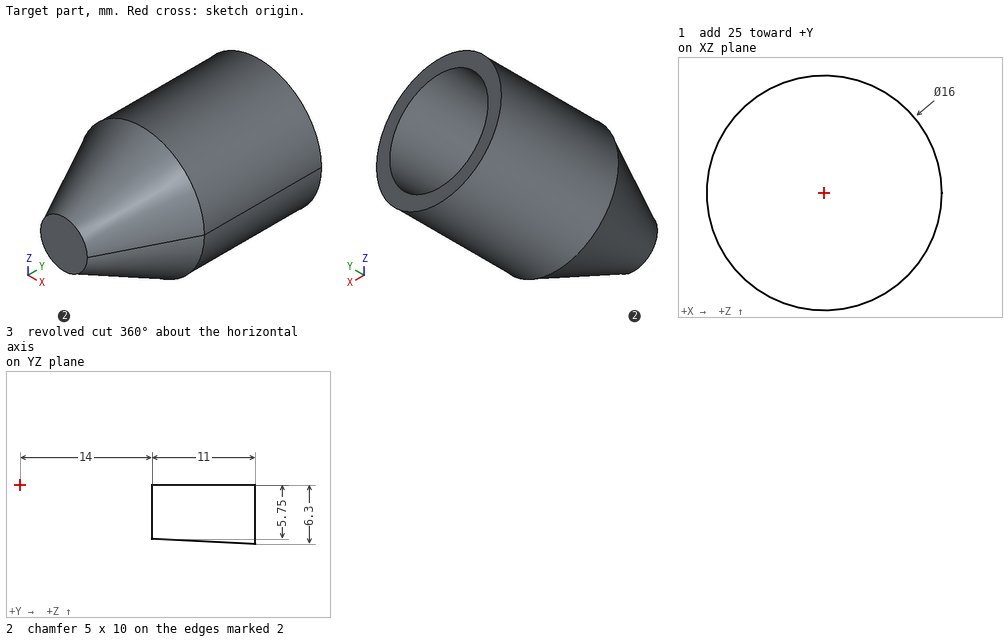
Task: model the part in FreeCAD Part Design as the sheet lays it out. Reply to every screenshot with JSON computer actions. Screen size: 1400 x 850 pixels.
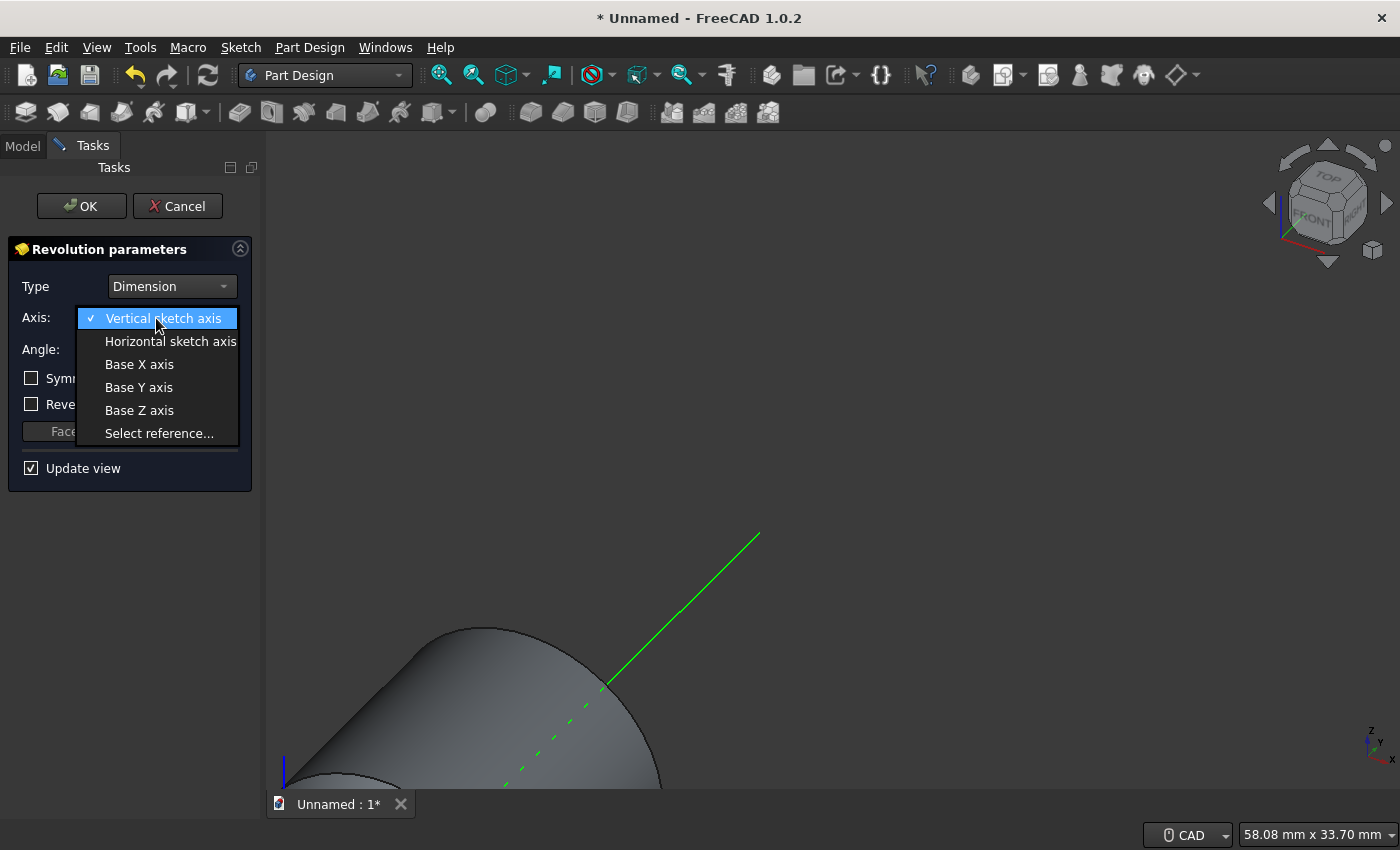
{"action": "left_click", "coordinate": [156, 342]}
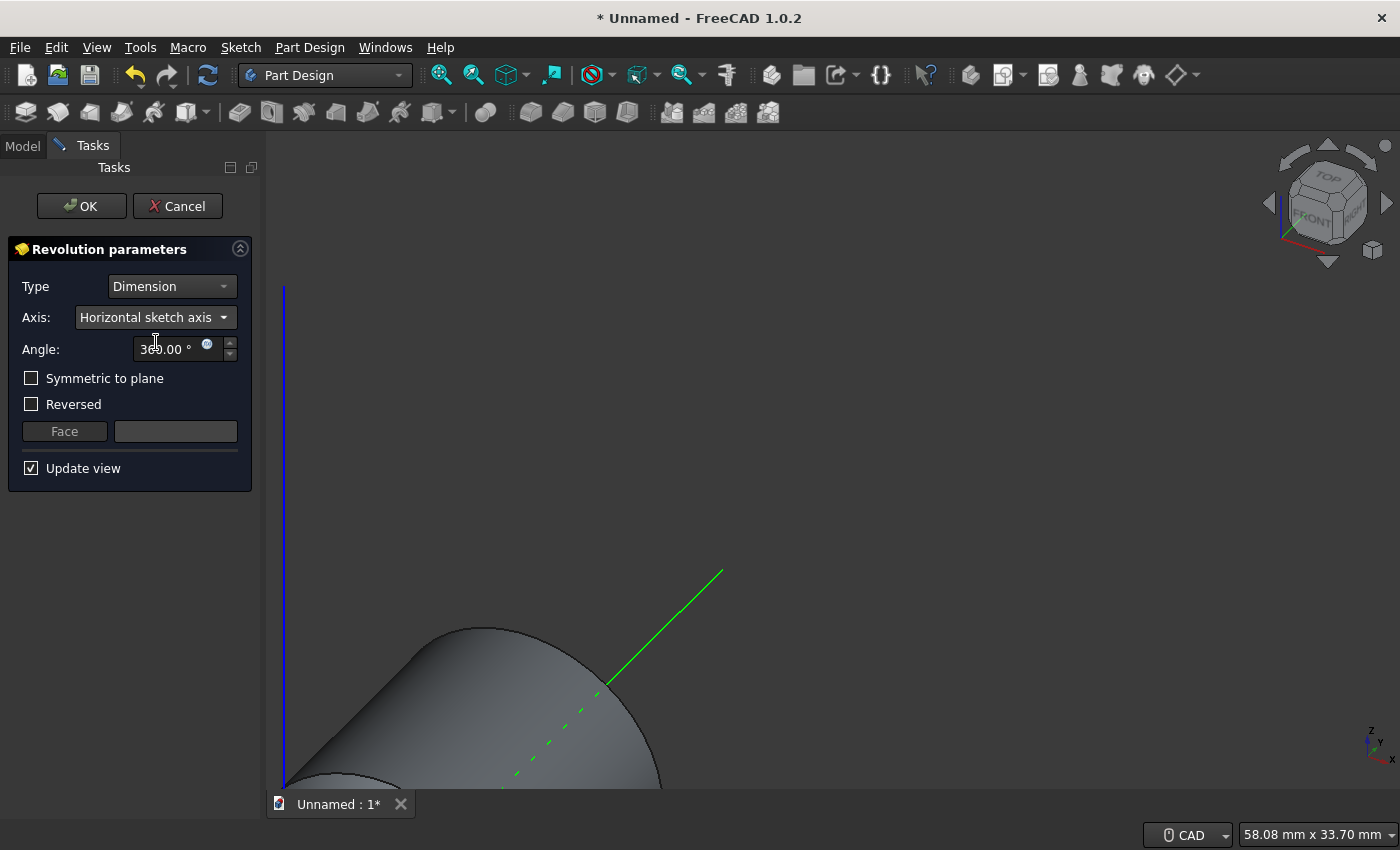
{"action": "left_click", "coordinate": [82, 206]}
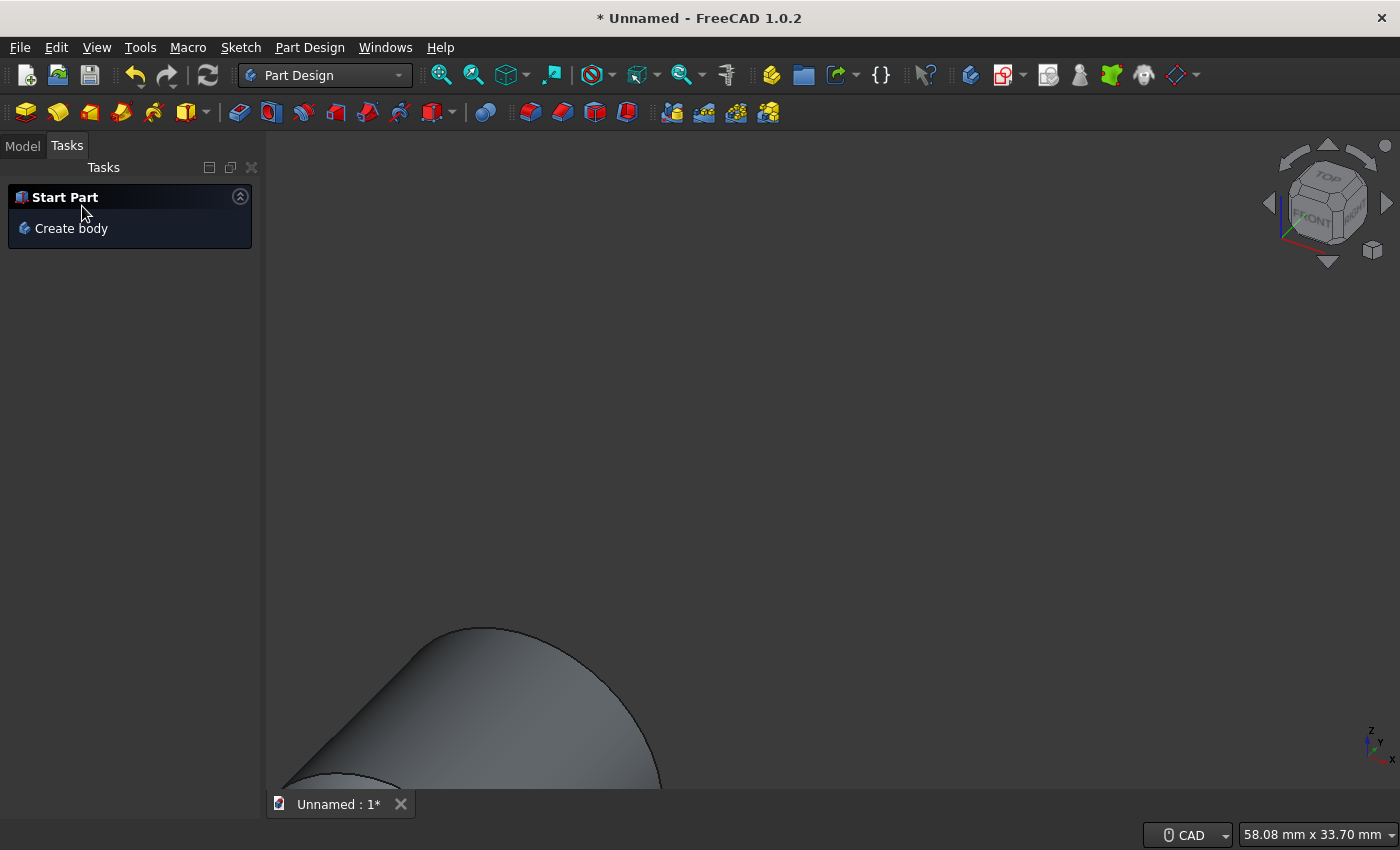
{"action": "key", "text": "0"}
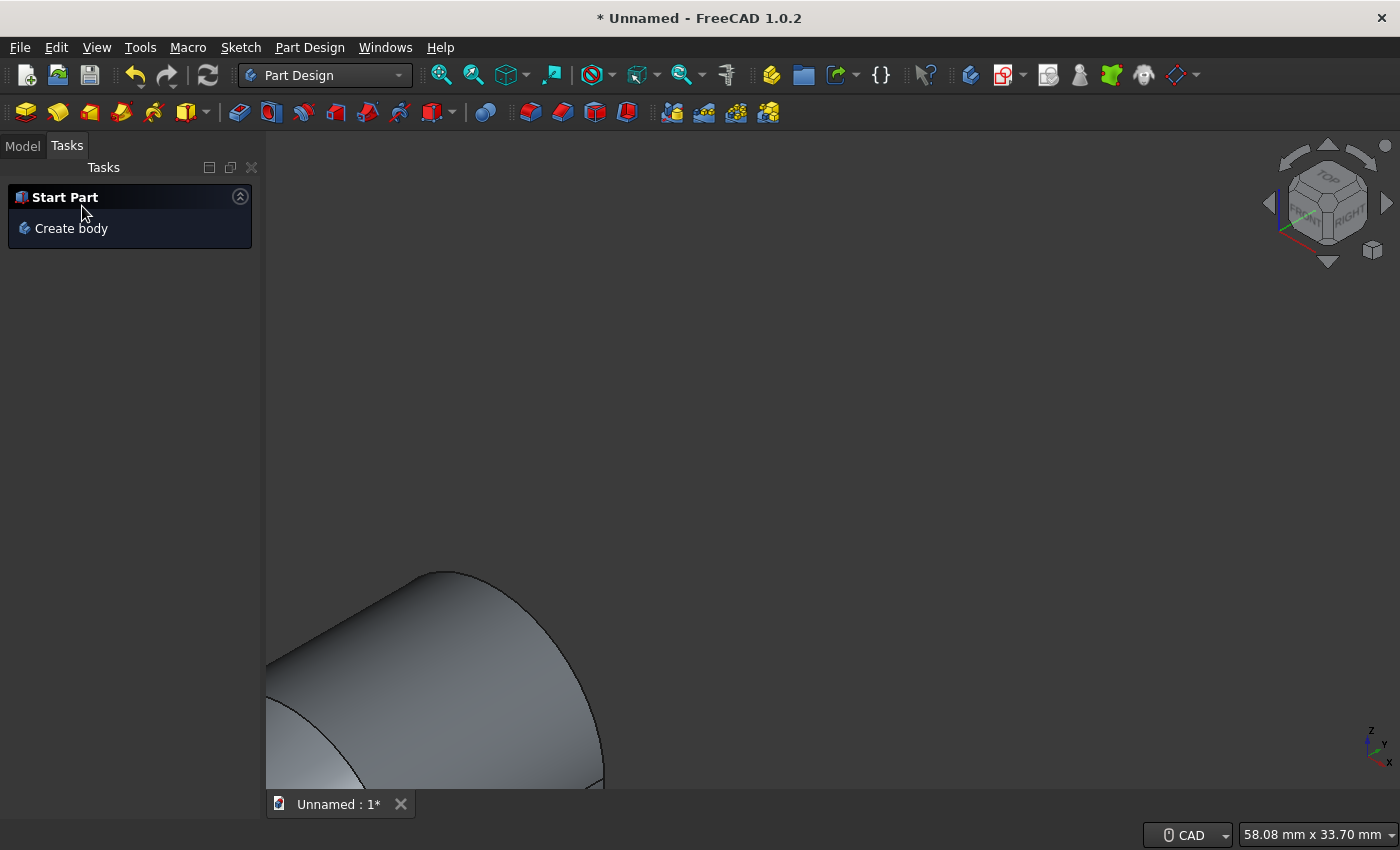
{"action": "left_click", "coordinate": [442, 76]}